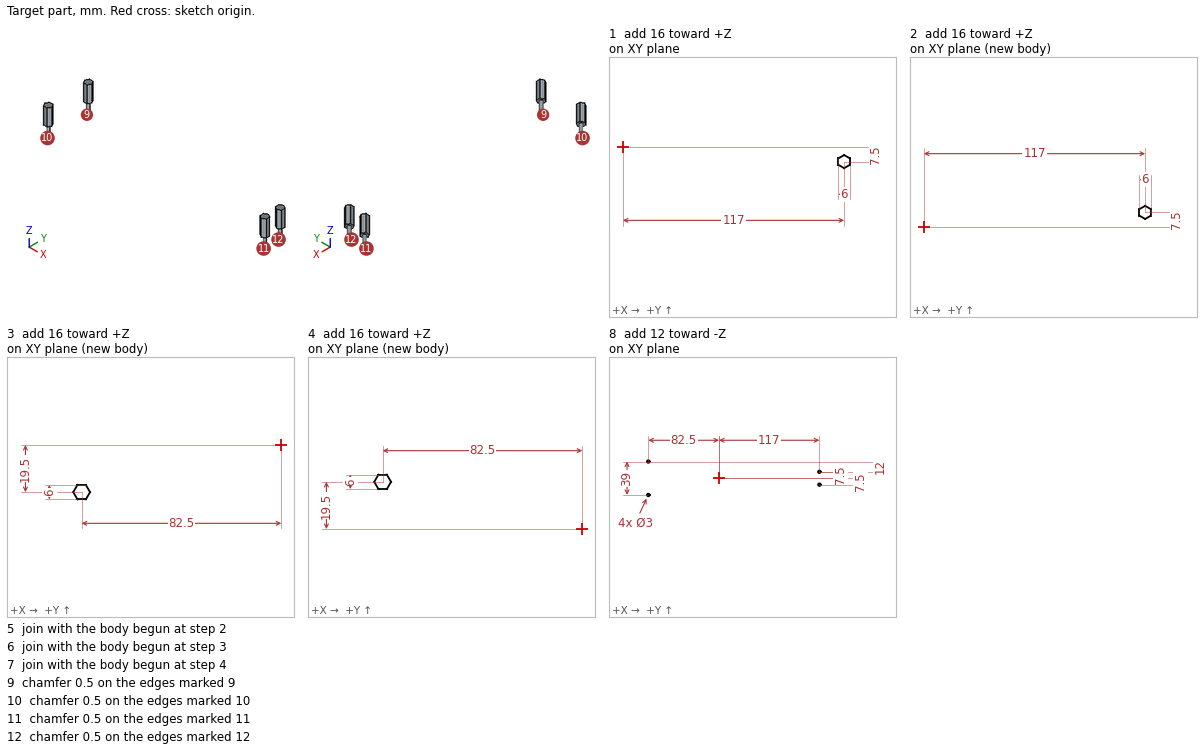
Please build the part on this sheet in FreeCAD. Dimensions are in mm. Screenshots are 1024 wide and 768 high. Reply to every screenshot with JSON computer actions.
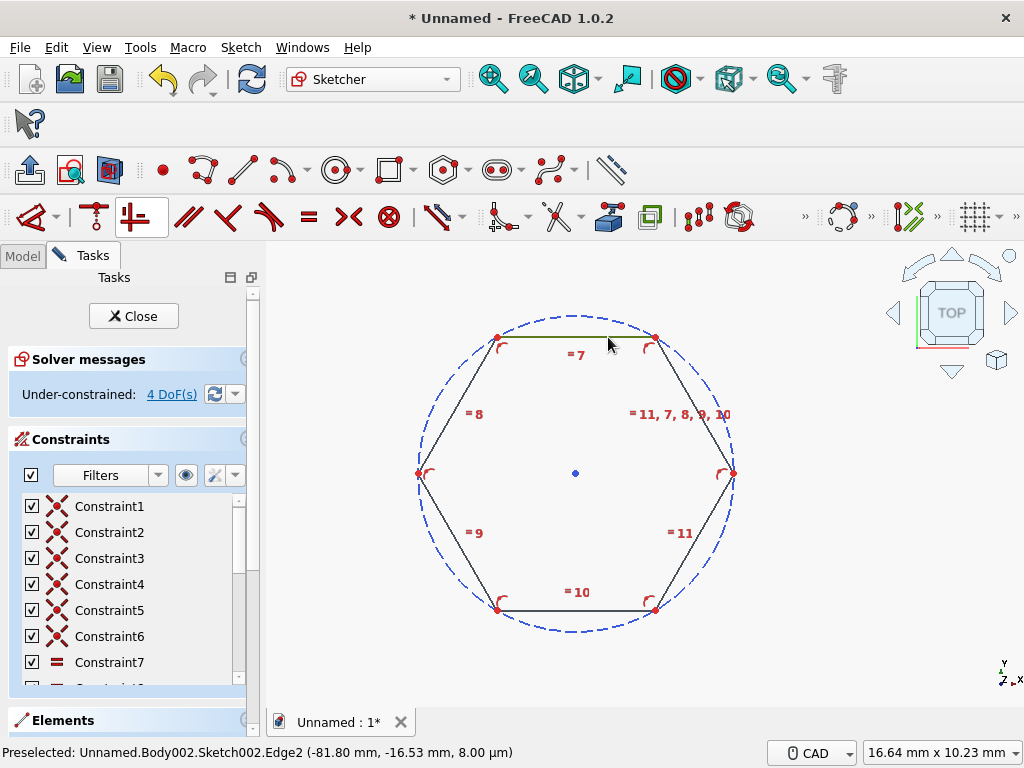
{"action": "left_click", "coordinate": [162, 218]}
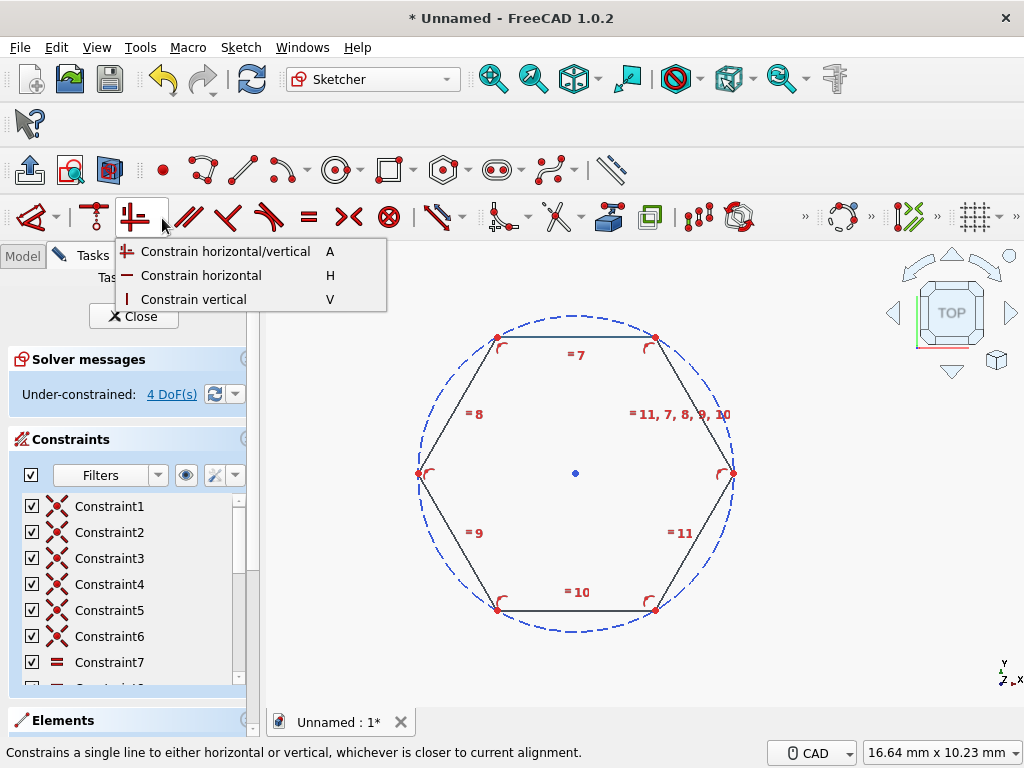
{"action": "left_click", "coordinate": [251, 275]}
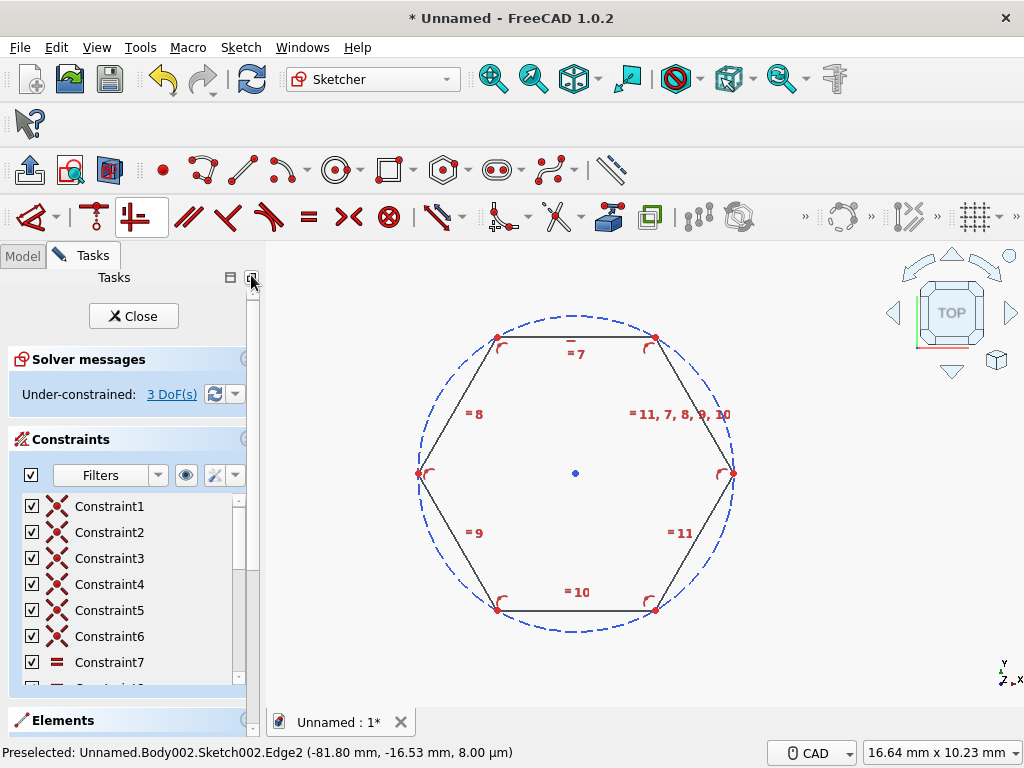
{"action": "left_click", "coordinate": [32, 218]}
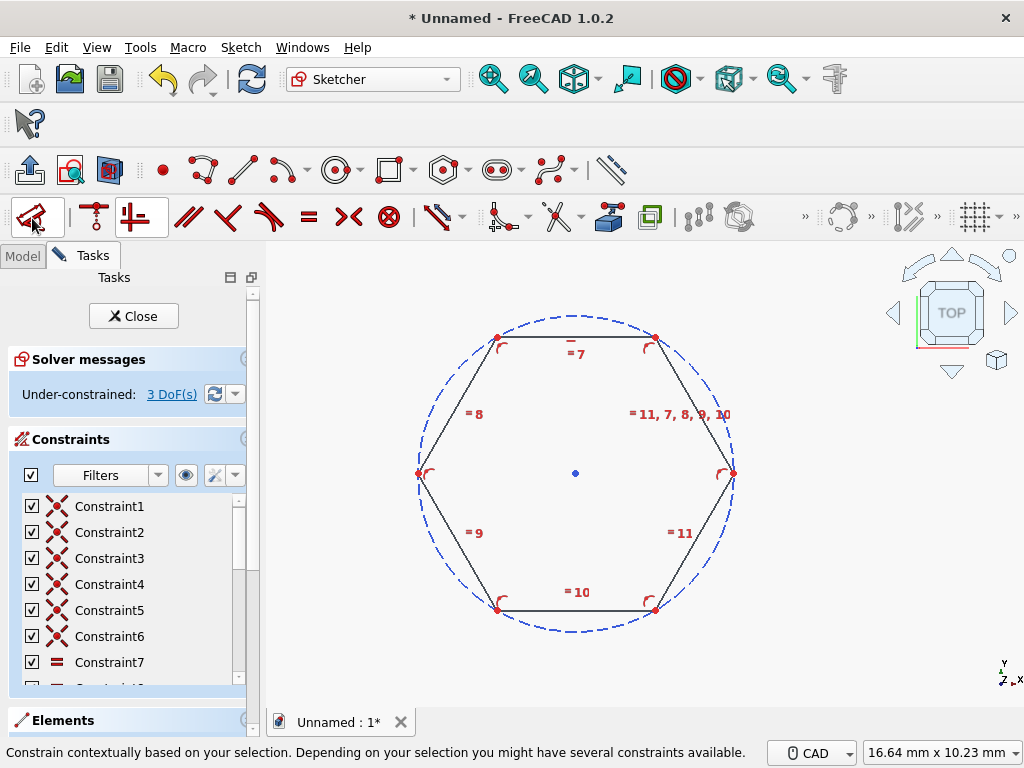
{"action": "left_click", "coordinate": [497, 611]}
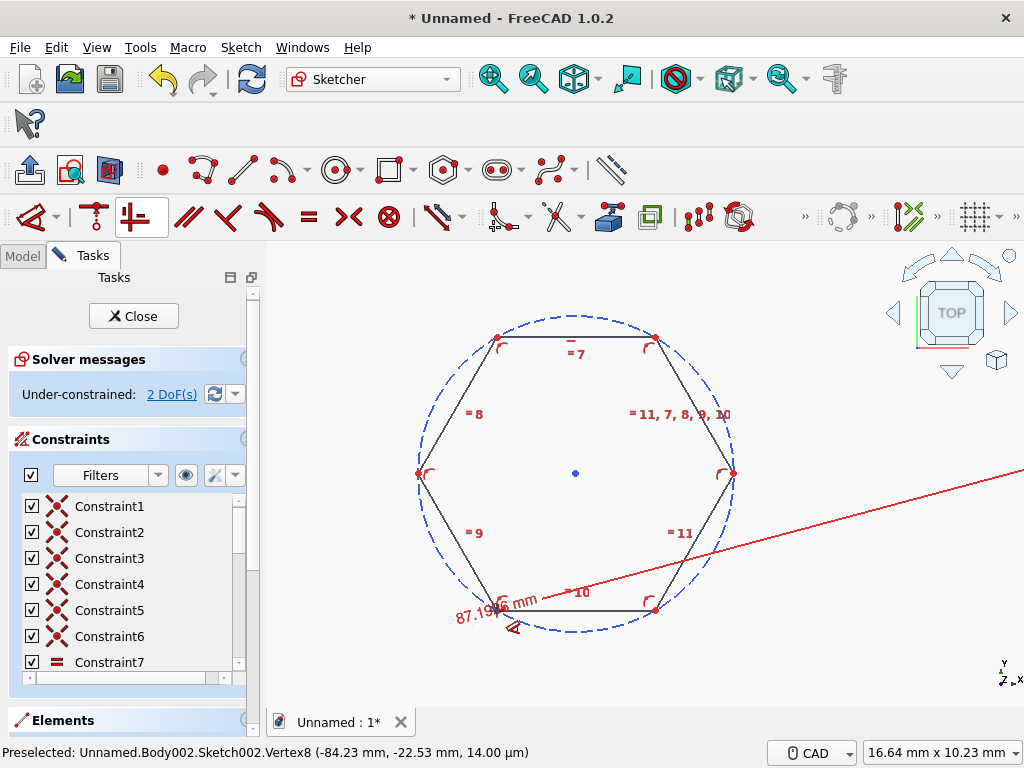
{"action": "left_click", "coordinate": [655, 337]}
{"action": "left_click", "coordinate": [689, 474]}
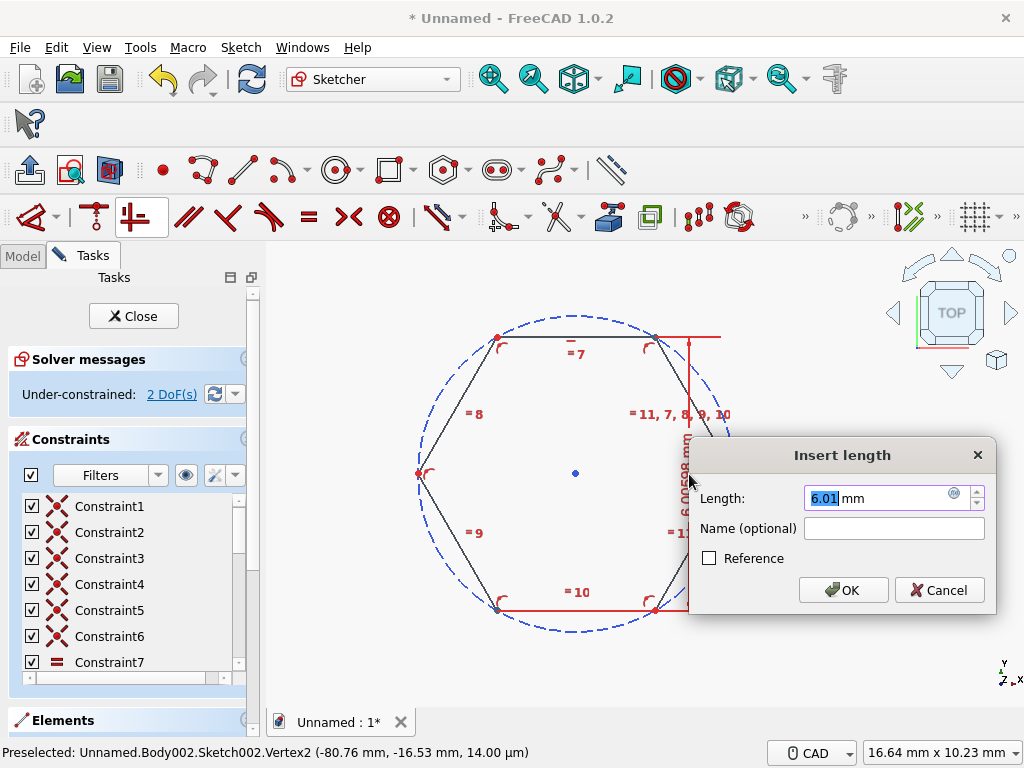
{"action": "type", "text": "6"}
{"action": "key", "text": "Return"}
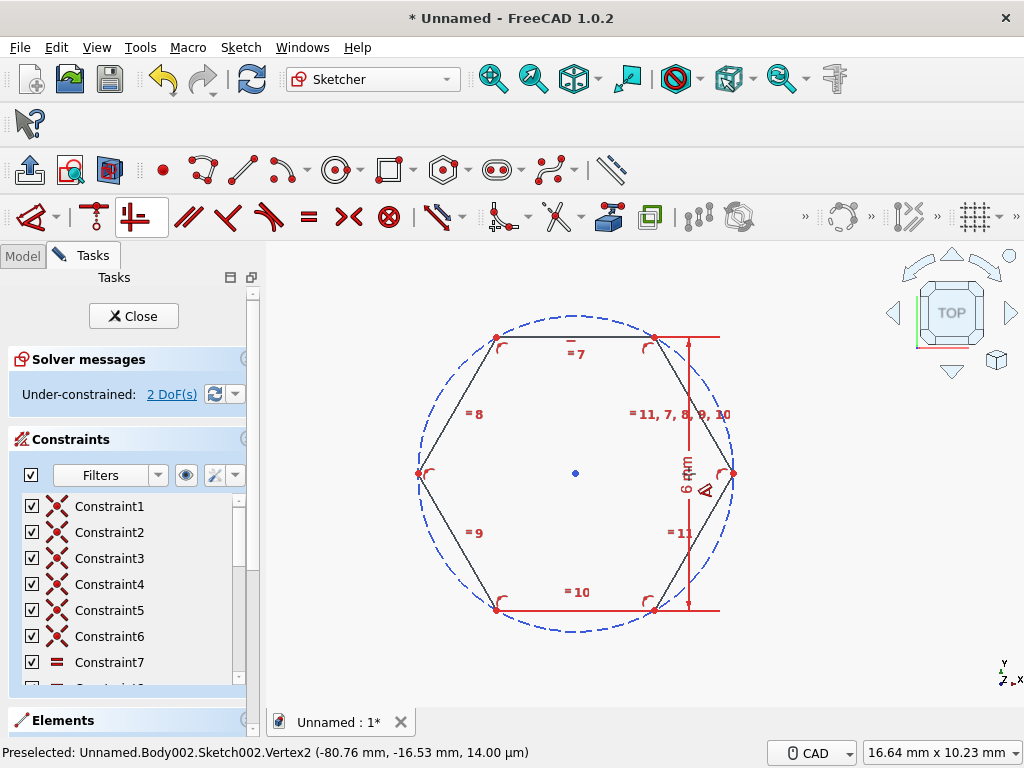
{"action": "left_click", "coordinate": [576, 474]}
{"action": "left_click", "coordinate": [652, 508]}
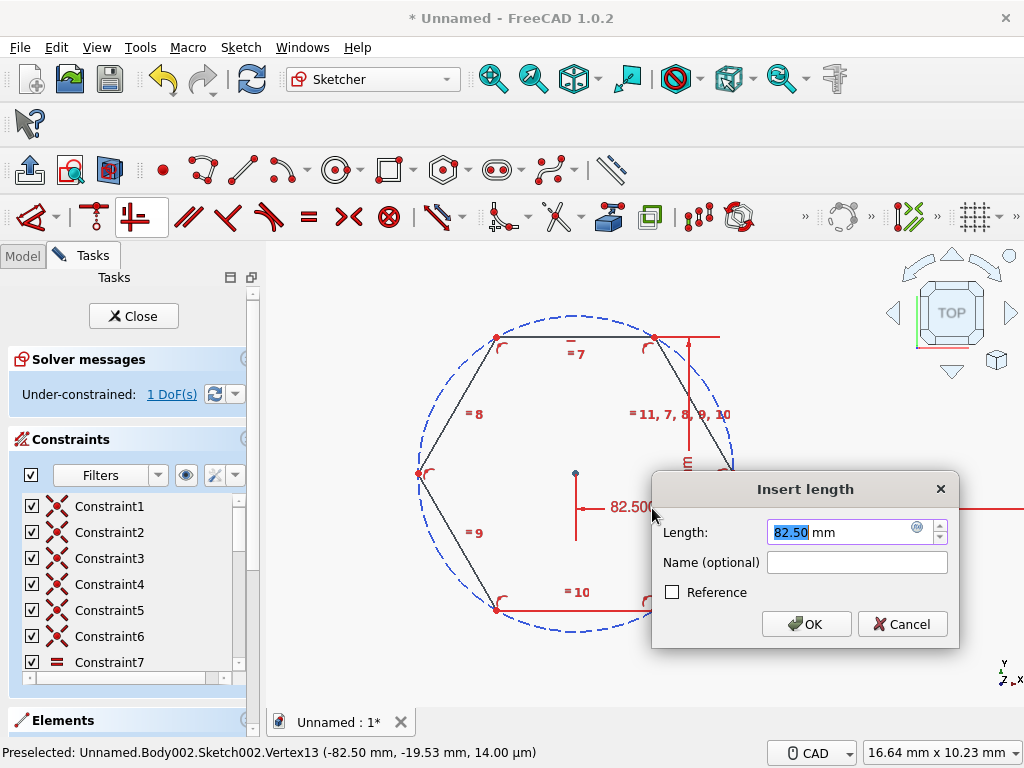
{"action": "type", "text": "82.5"}
{"action": "key", "text": "Return"}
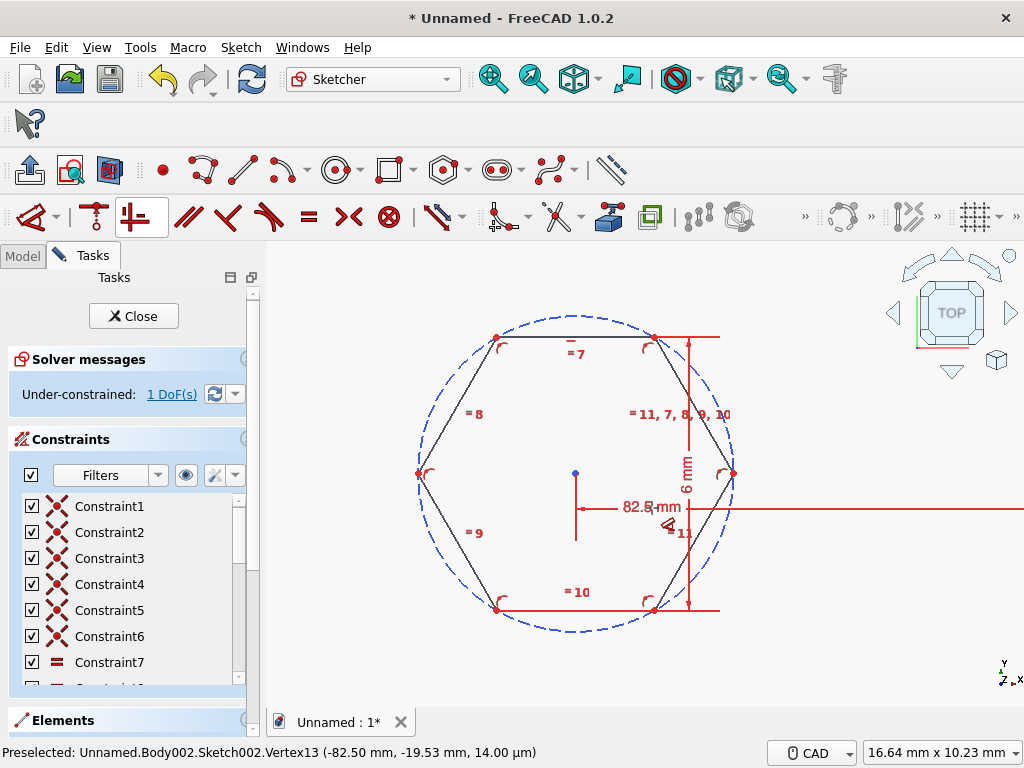
{"action": "left_click", "coordinate": [576, 474]}
{"action": "left_click", "coordinate": [542, 372]}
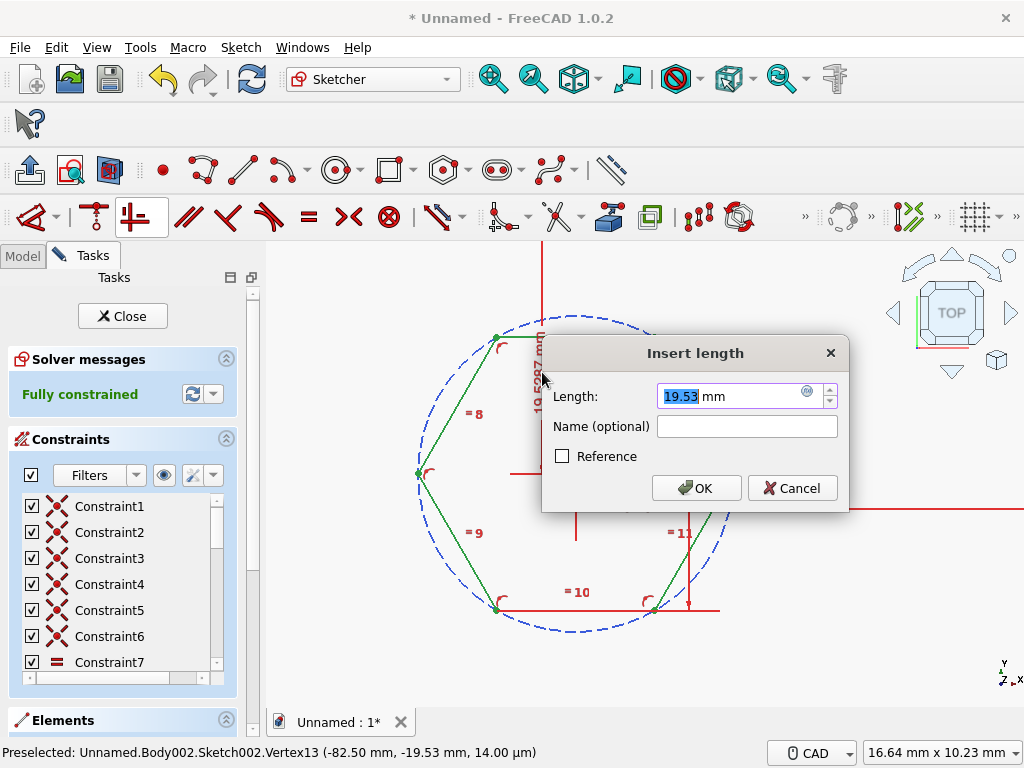
{"action": "type", "text": "19.5"}
{"action": "key", "text": "Return"}
{"action": "key", "text": "Escape"}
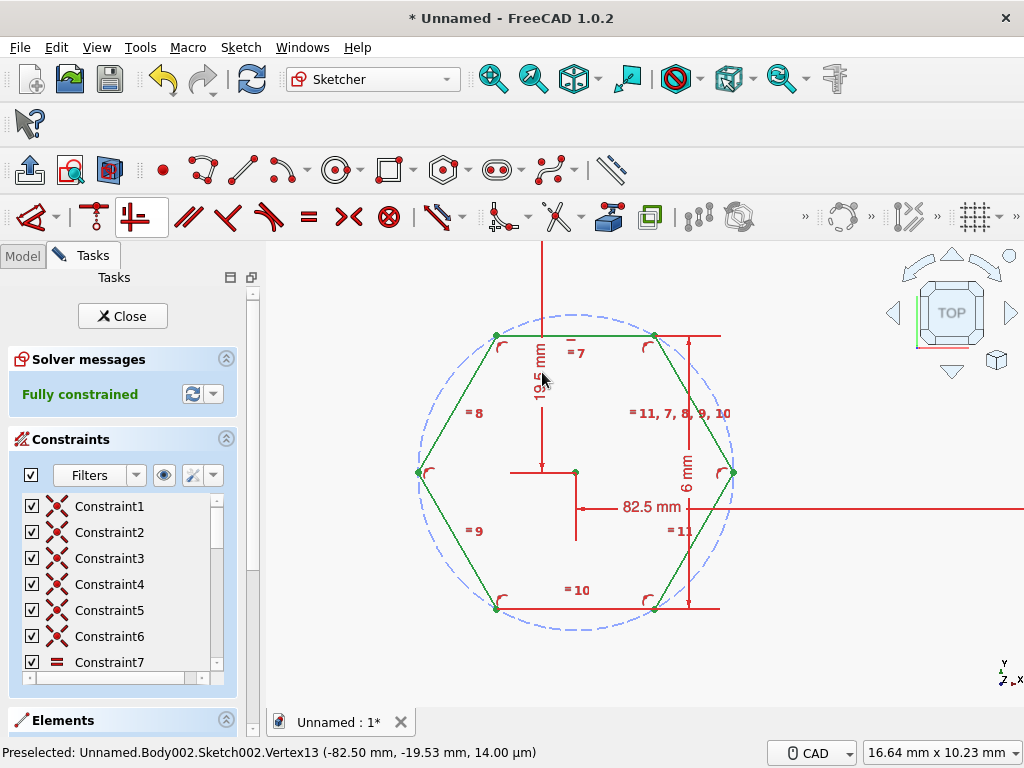
{"action": "left_click", "coordinate": [123, 316]}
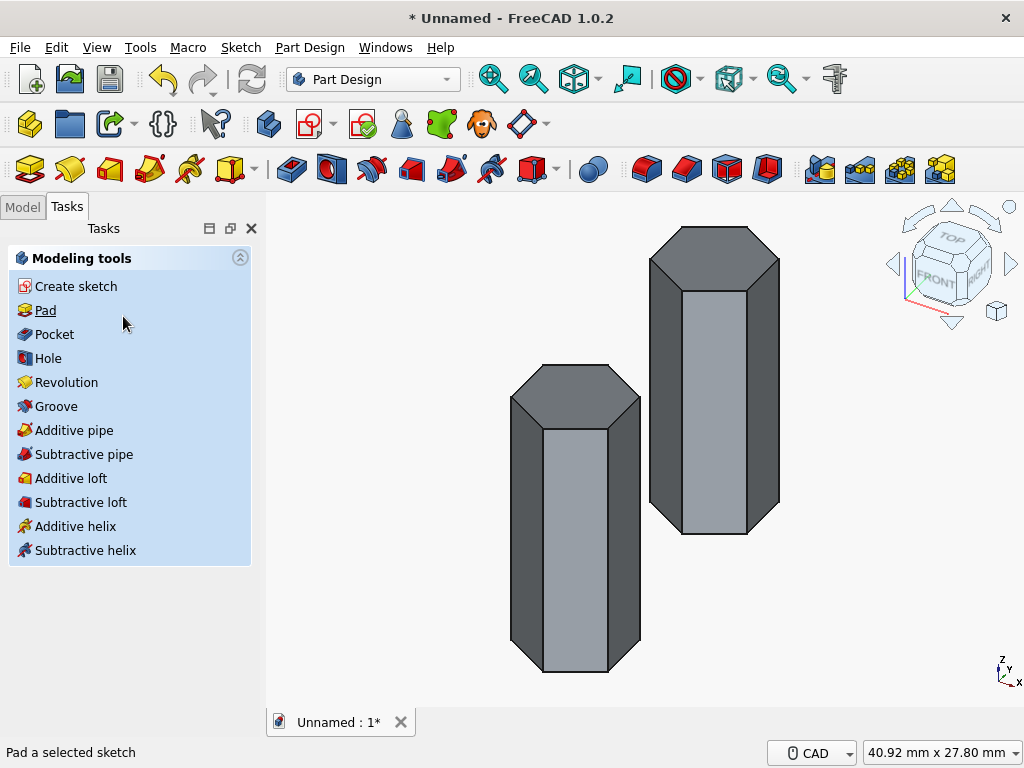
{"action": "left_click", "coordinate": [30, 170]}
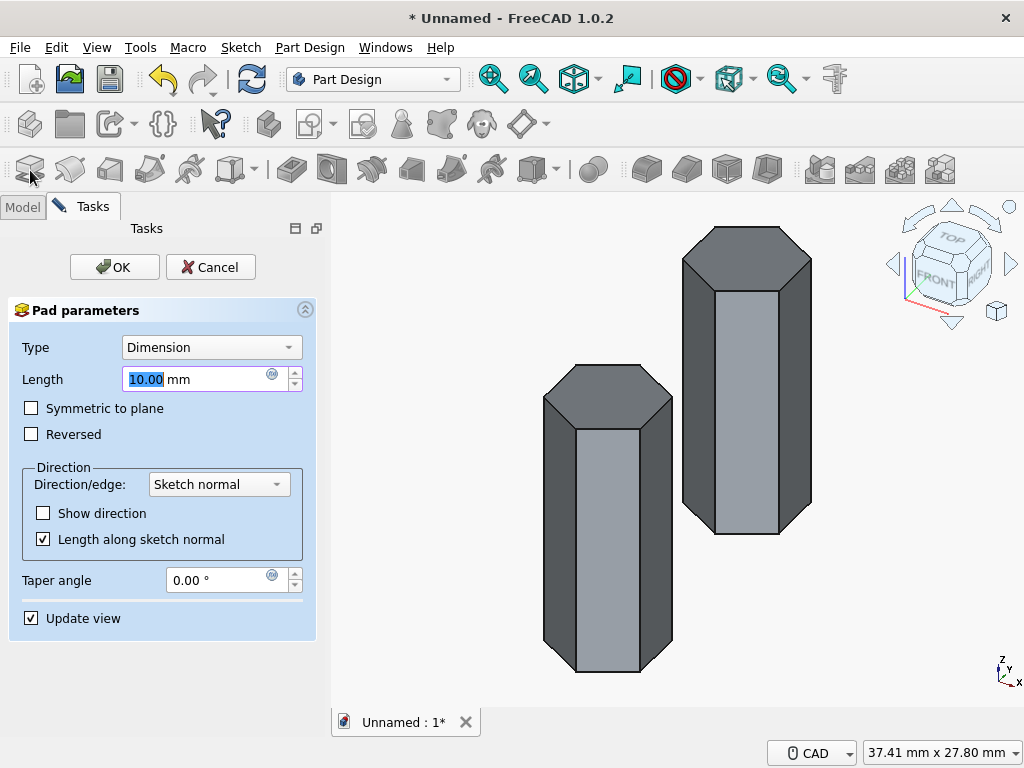
{"action": "type", "text": "16"}
{"action": "key", "text": "Tab"}